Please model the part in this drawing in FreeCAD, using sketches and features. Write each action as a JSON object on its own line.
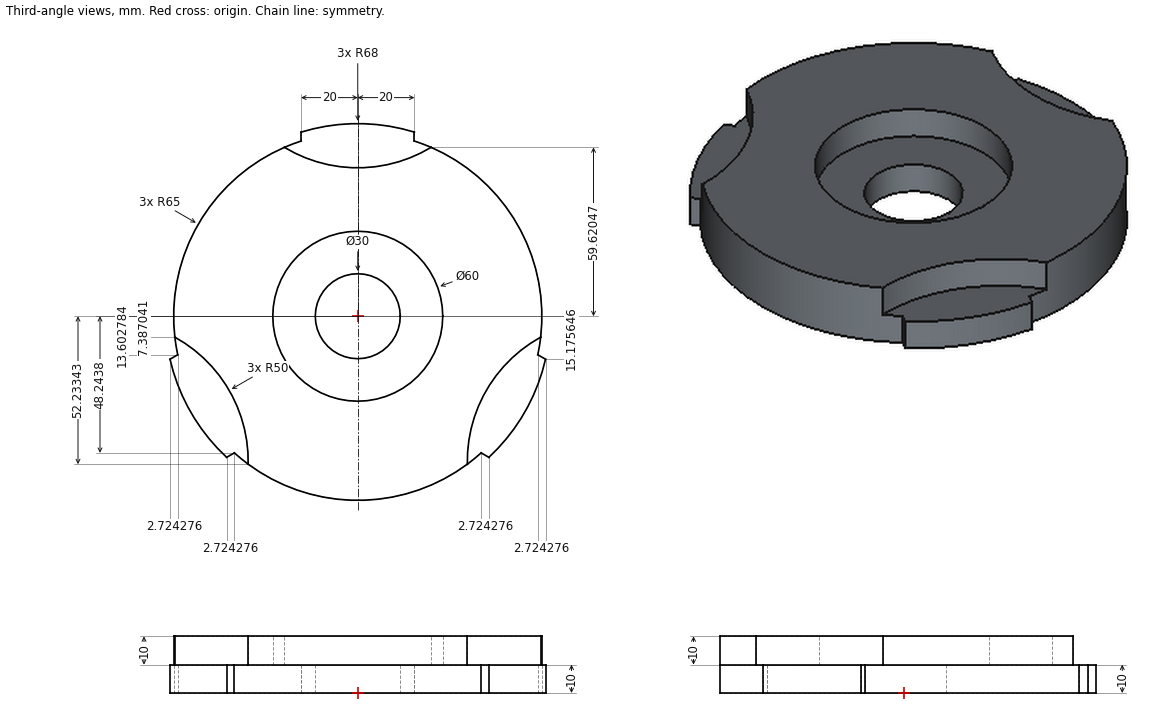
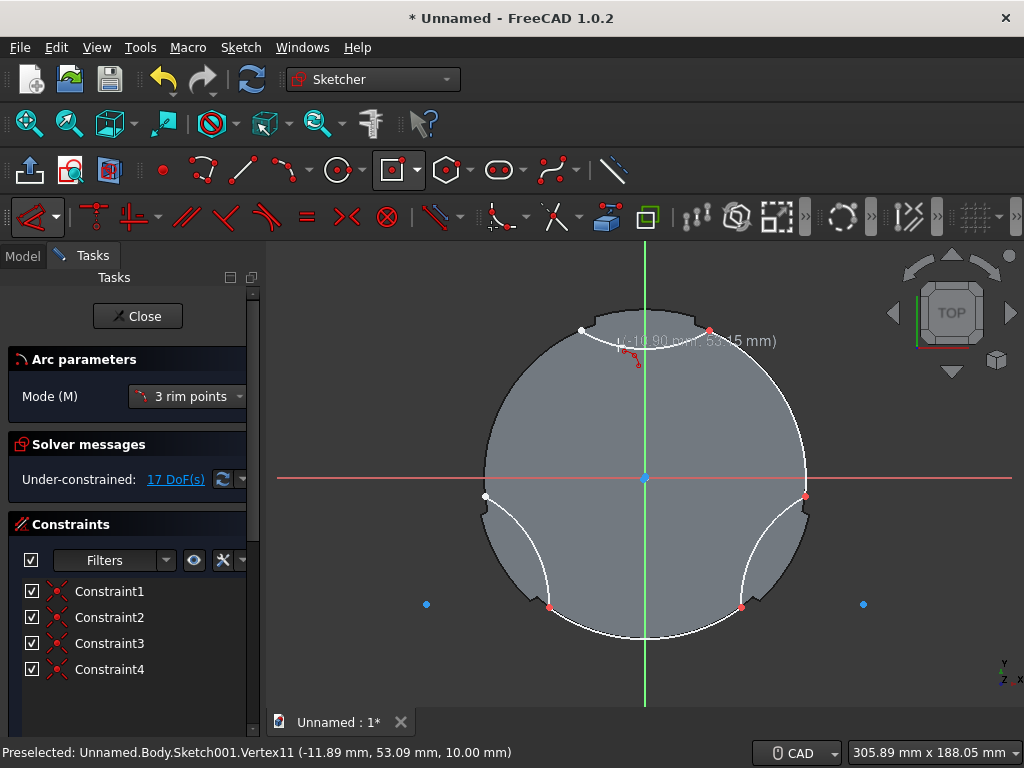
{"action": "left_click", "coordinate": [581, 331]}
{"action": "left_click", "coordinate": [485, 497]}
{"action": "left_click", "coordinate": [506, 397]}
{"action": "key", "text": "Escape"}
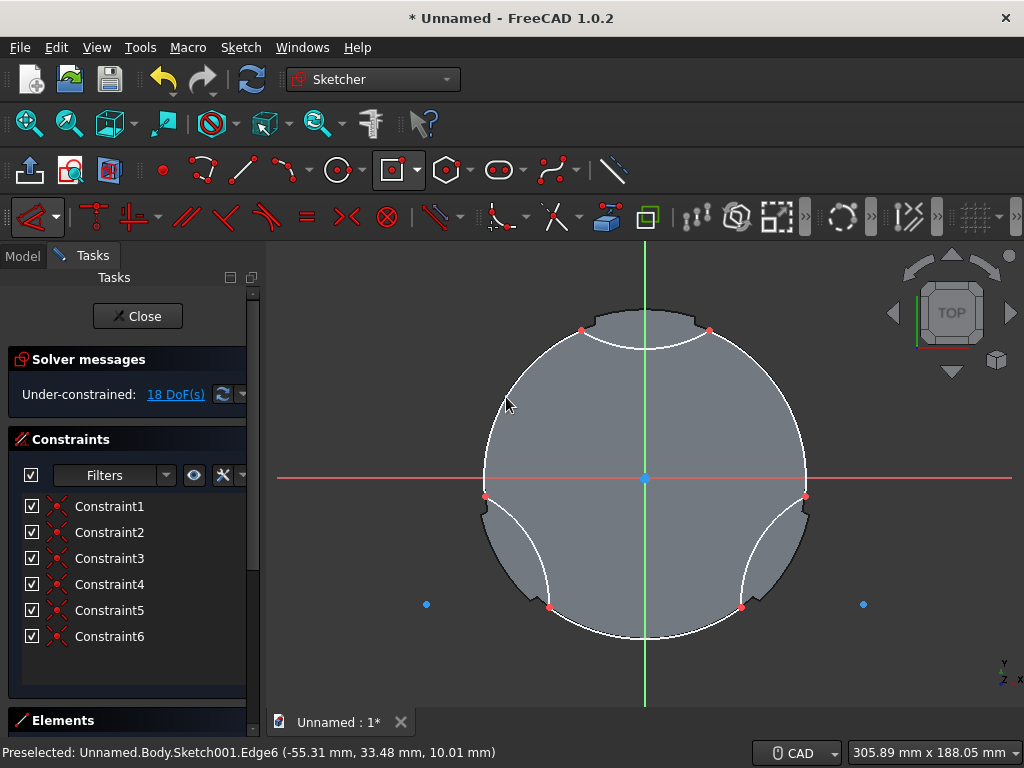
{"action": "left_click", "coordinate": [604, 634]}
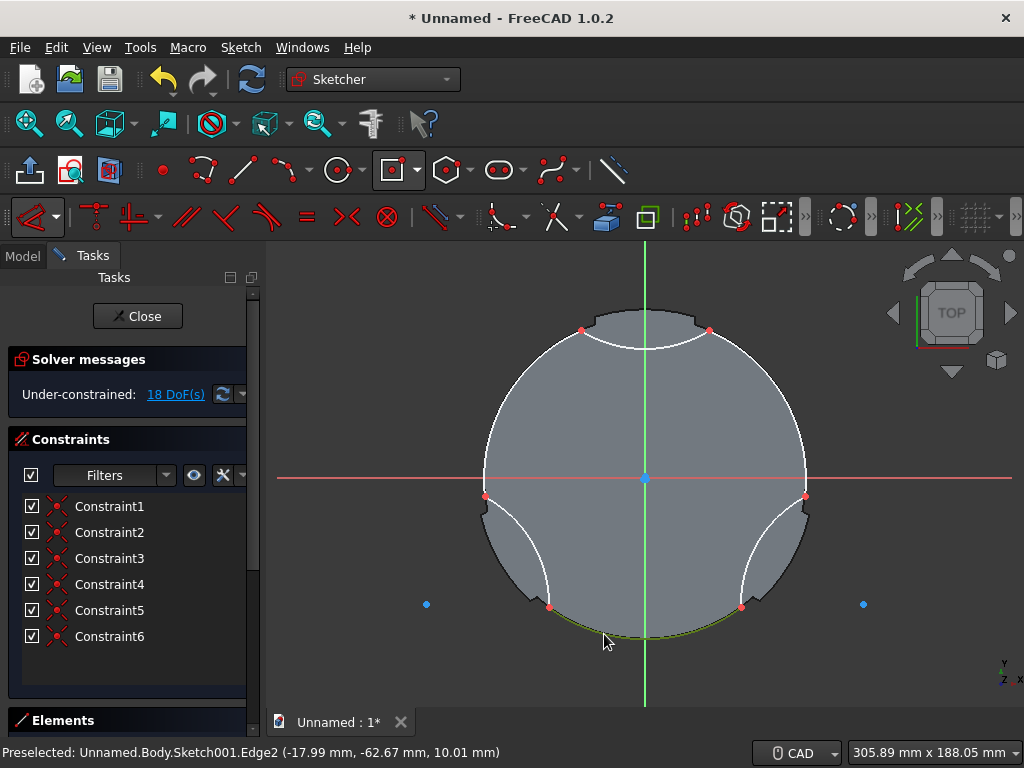
{"action": "left_click", "coordinate": [800, 436]}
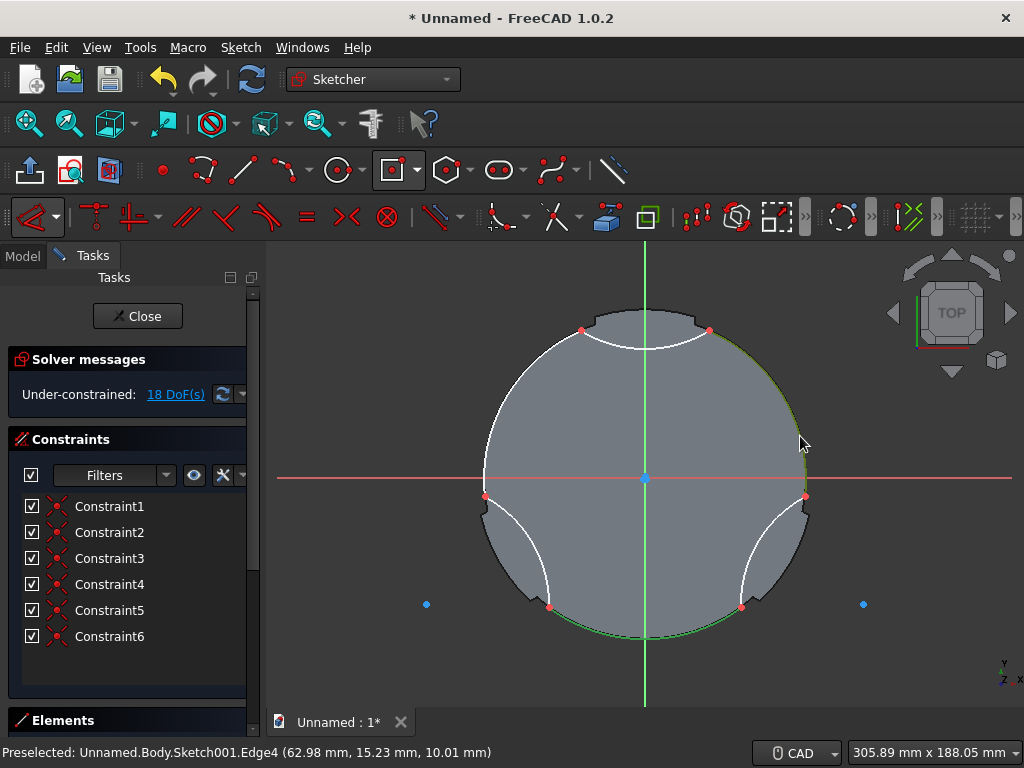
{"action": "left_click", "coordinate": [94, 218]}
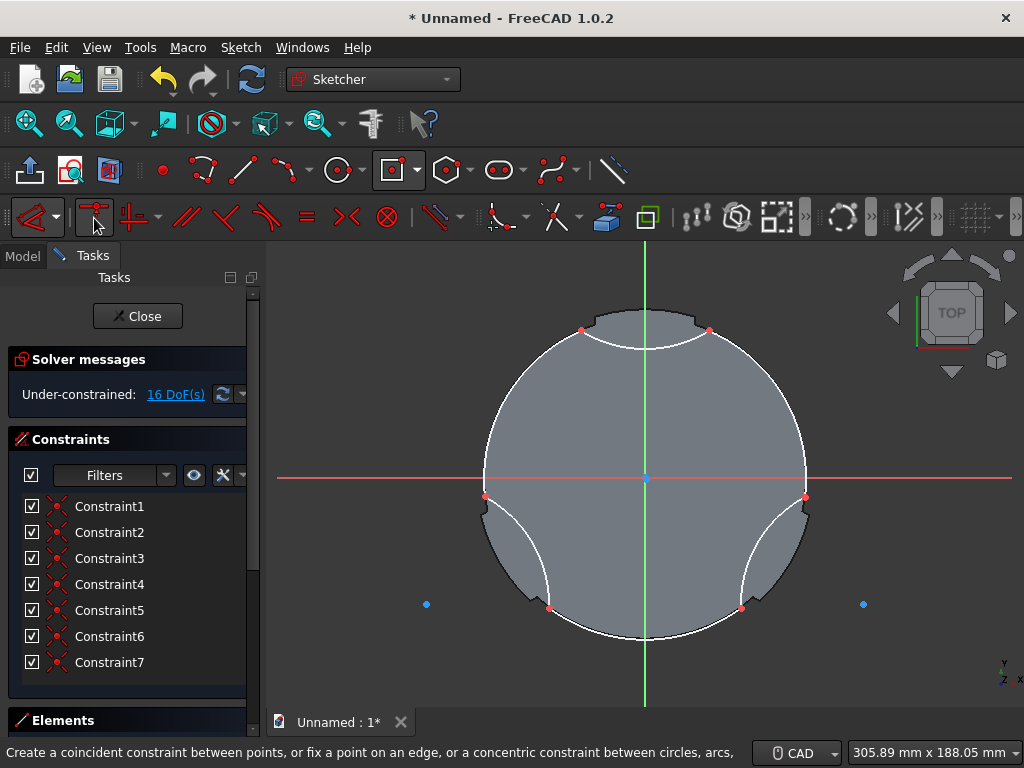
{"action": "left_click", "coordinate": [604, 635]}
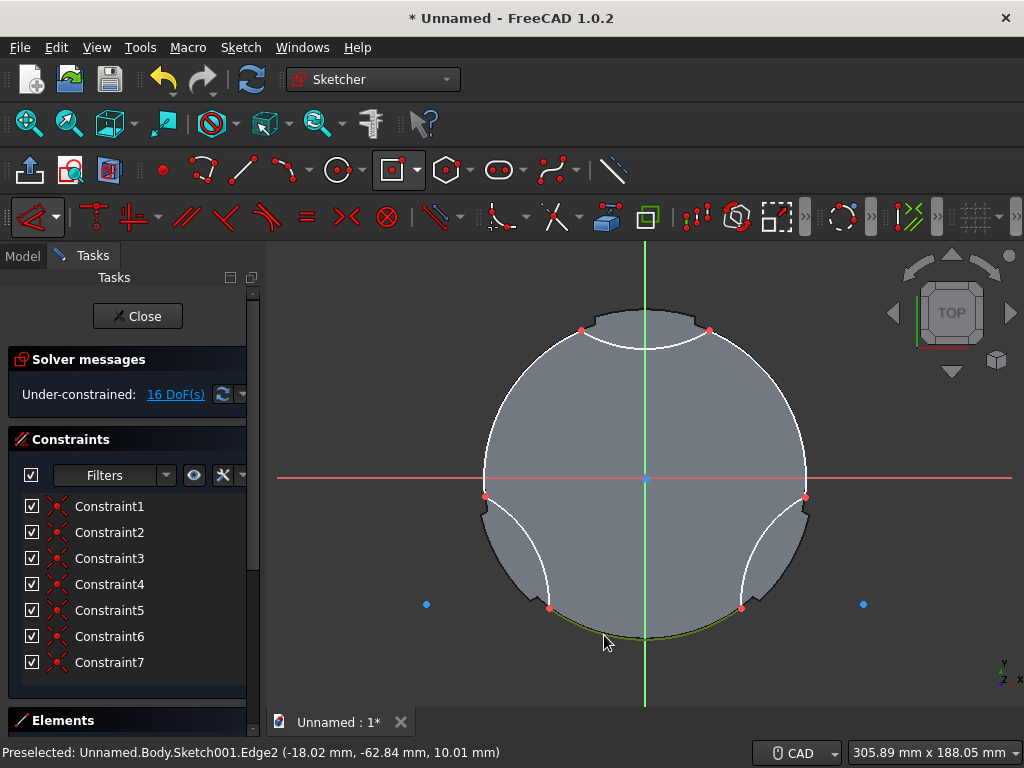
{"action": "left_click", "coordinate": [531, 366]}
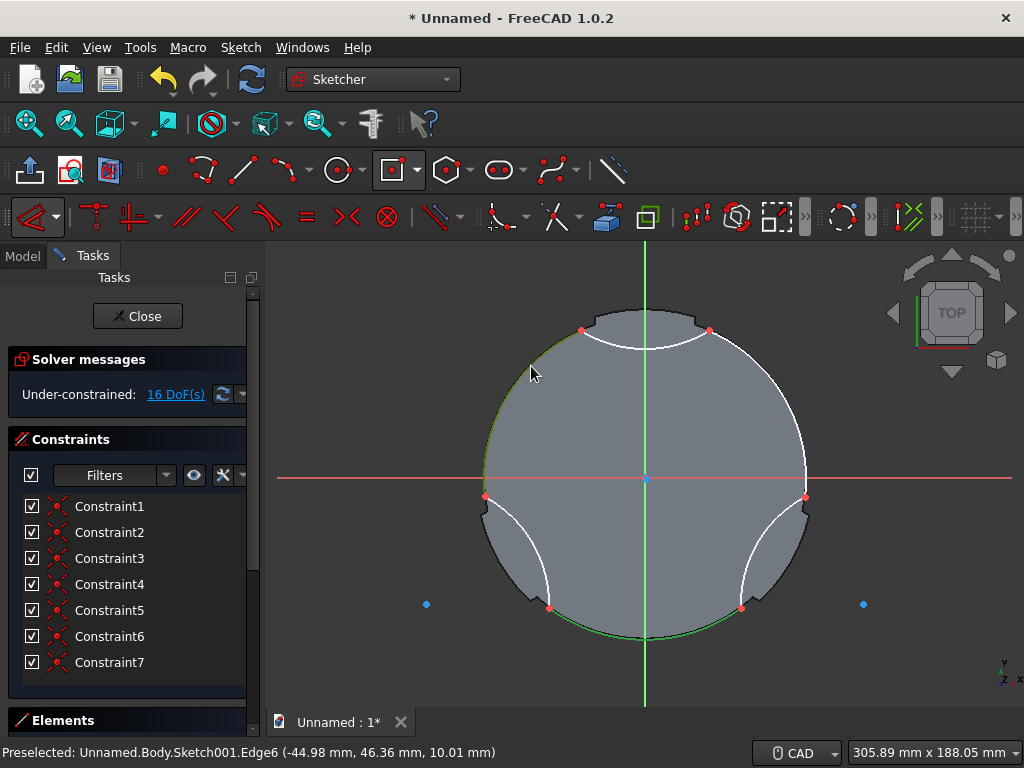
{"action": "left_click", "coordinate": [94, 218]}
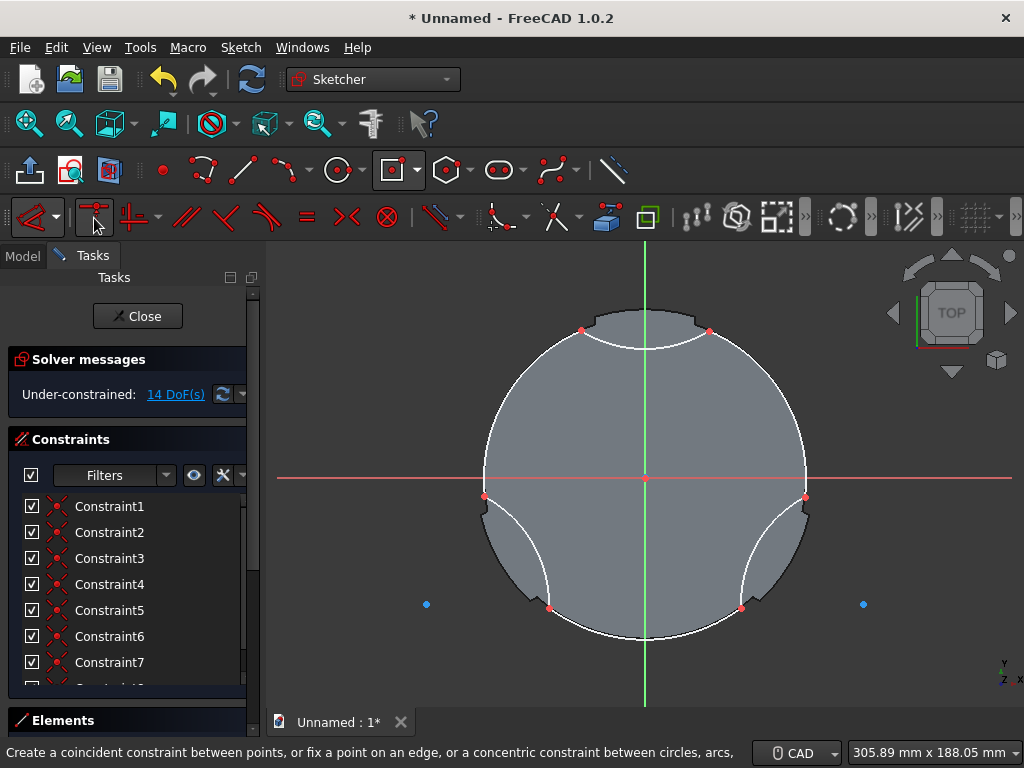
{"action": "left_click_drag", "start_coordinate": [635, 468], "coordinate": [655, 489]}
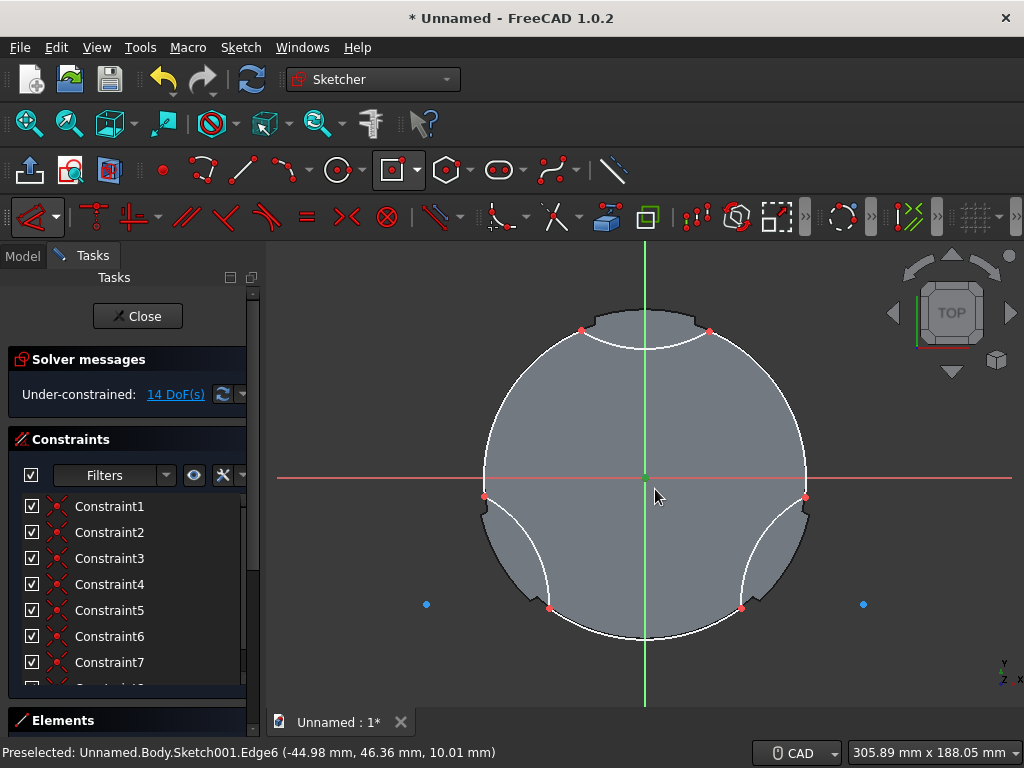
{"action": "left_click", "coordinate": [94, 218]}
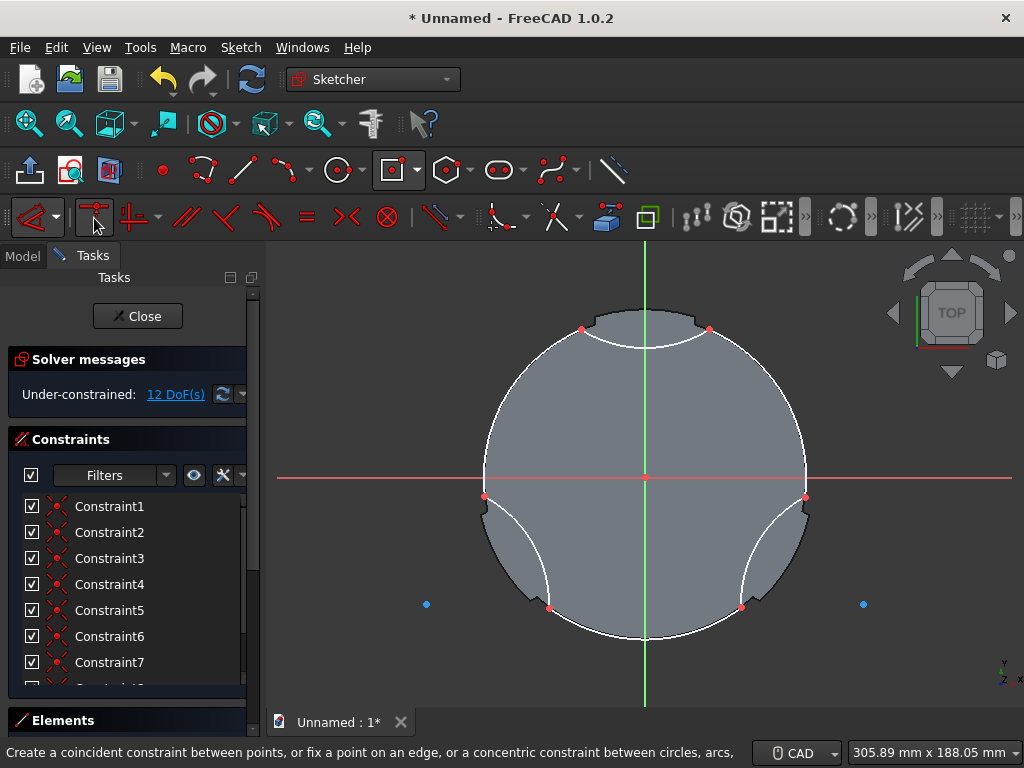
{"action": "left_click", "coordinate": [543, 568]}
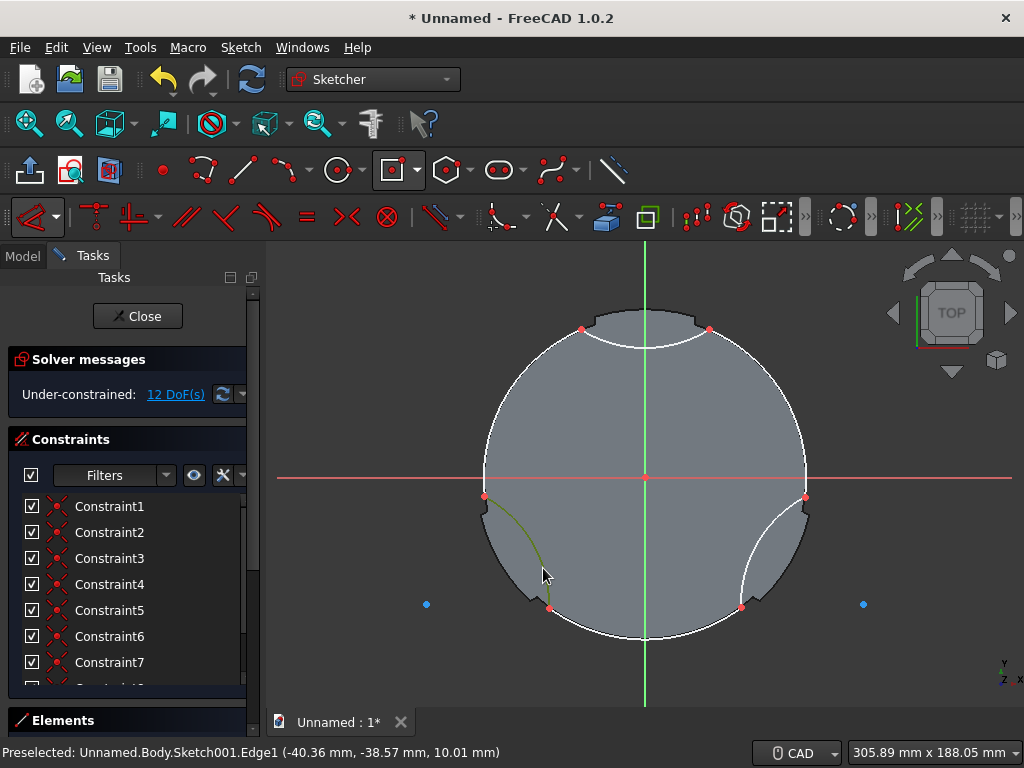
{"action": "left_click", "coordinate": [773, 522]}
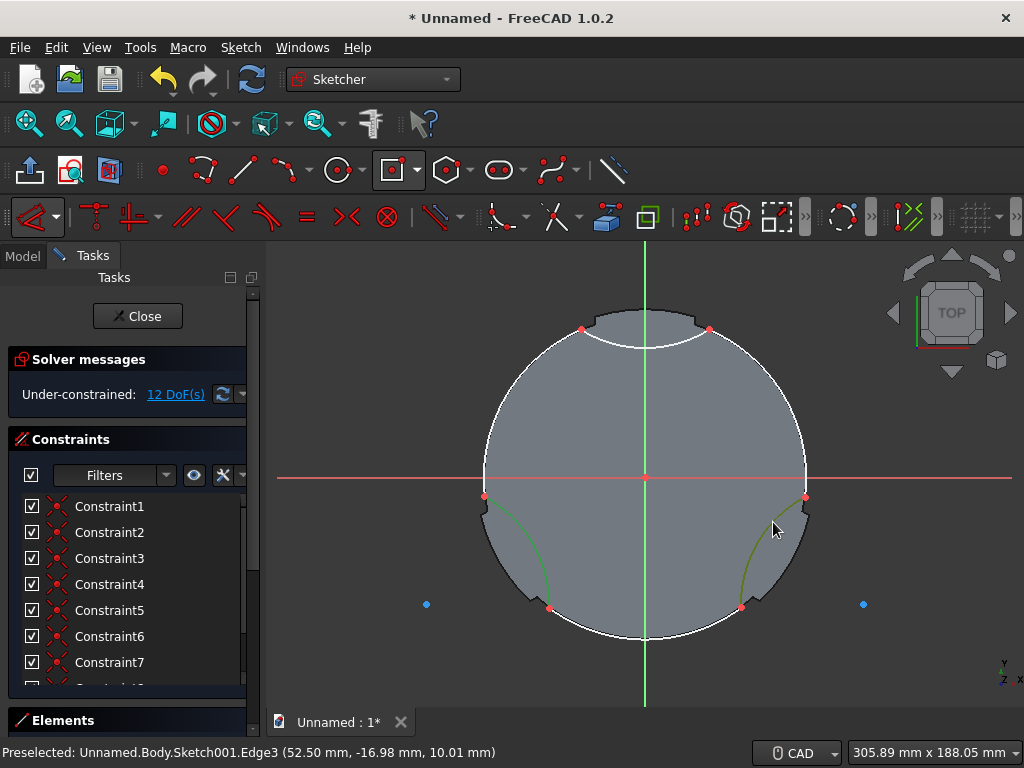
{"action": "left_click", "coordinate": [618, 345]}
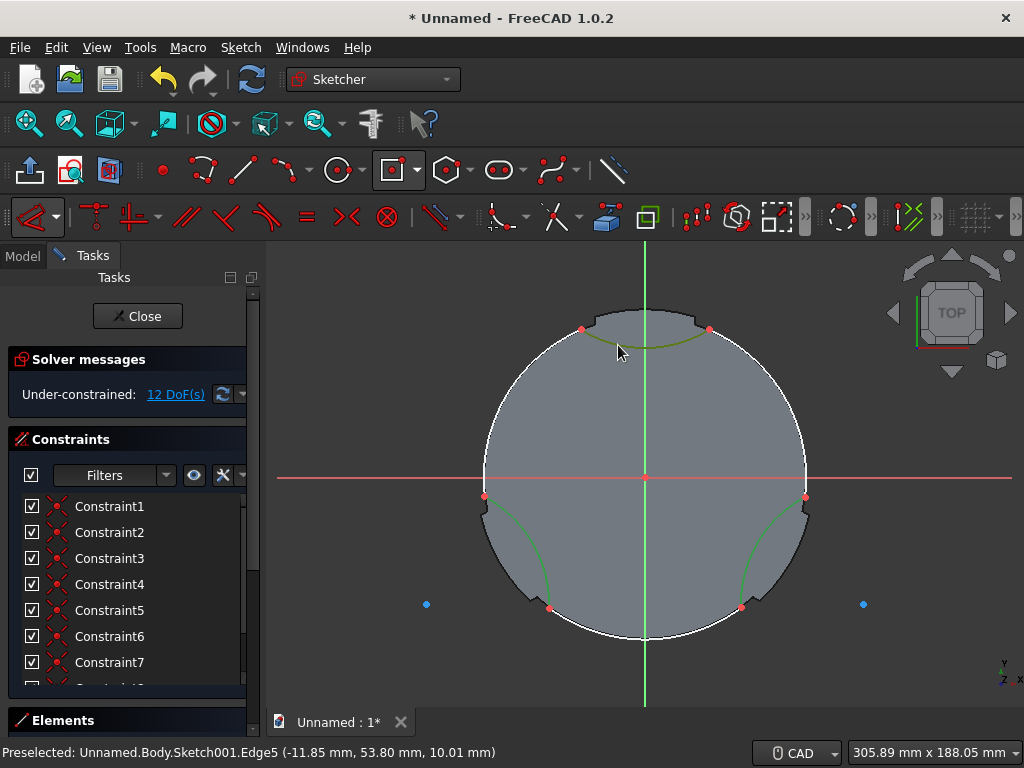
{"action": "left_click", "coordinate": [308, 218]}